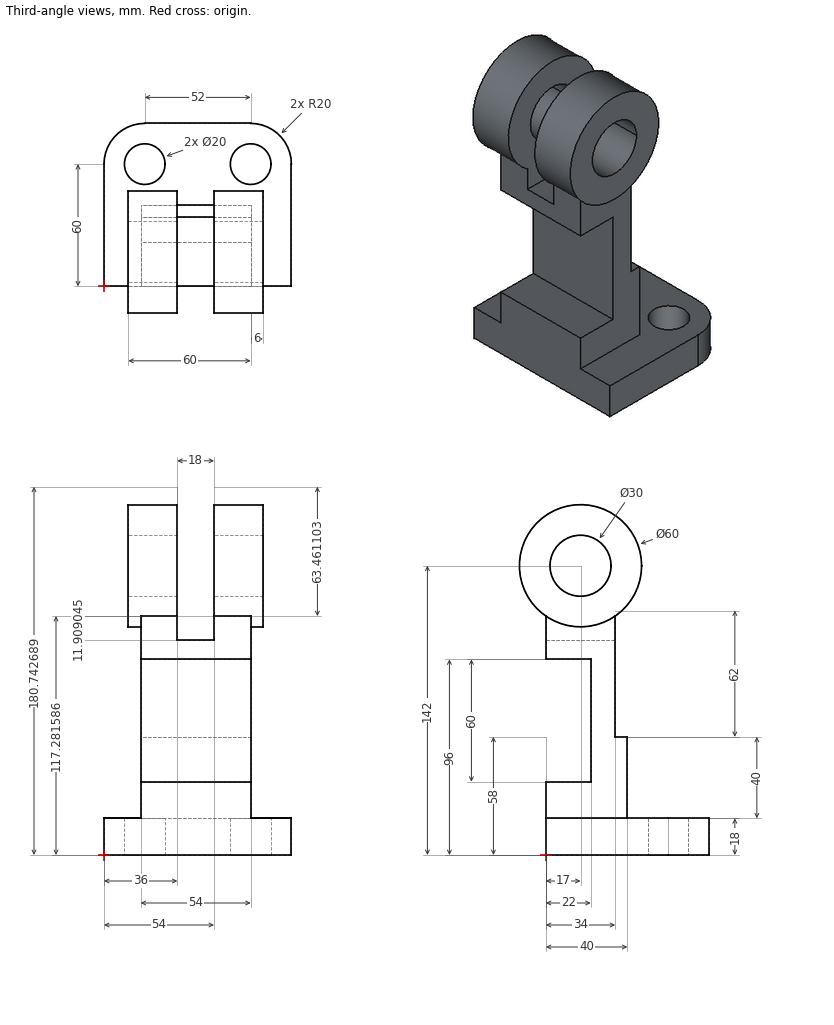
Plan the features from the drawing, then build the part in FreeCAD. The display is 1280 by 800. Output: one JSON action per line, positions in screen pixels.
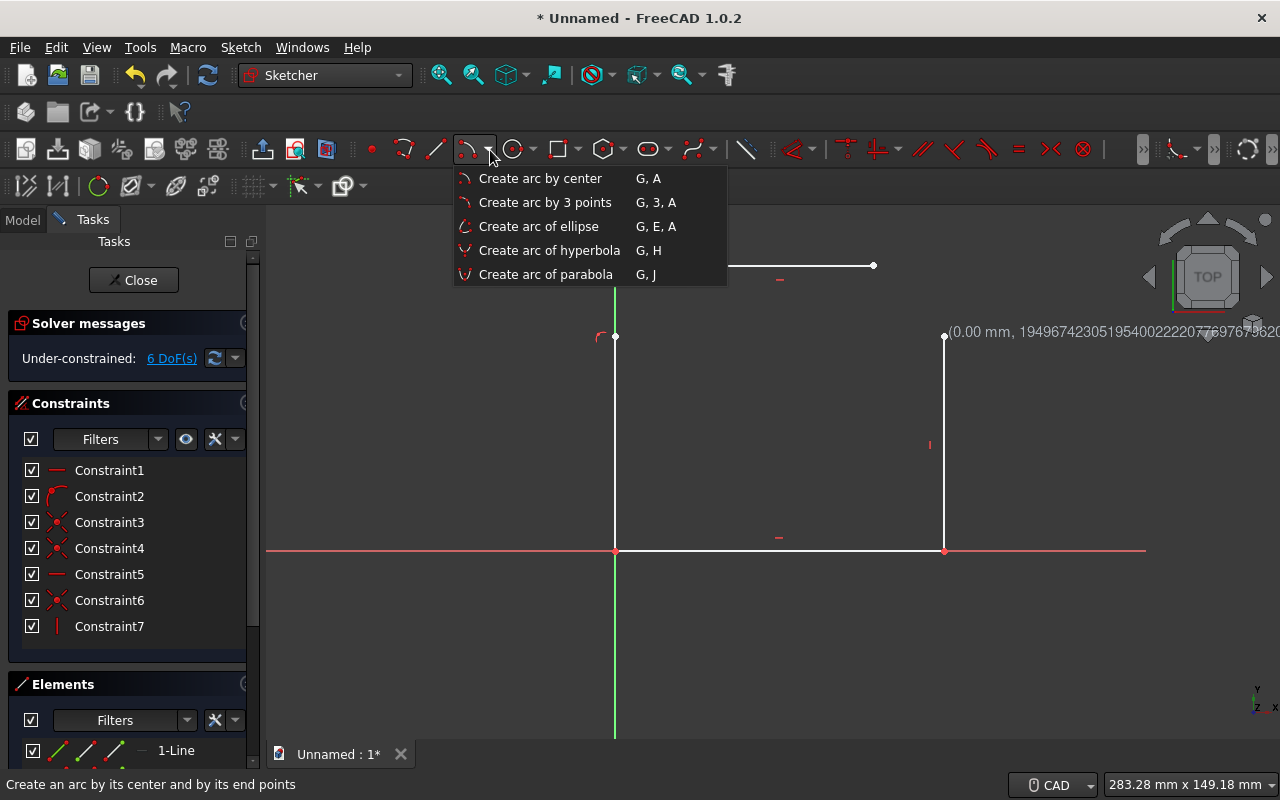
{"action": "left_click", "coordinate": [590, 202]}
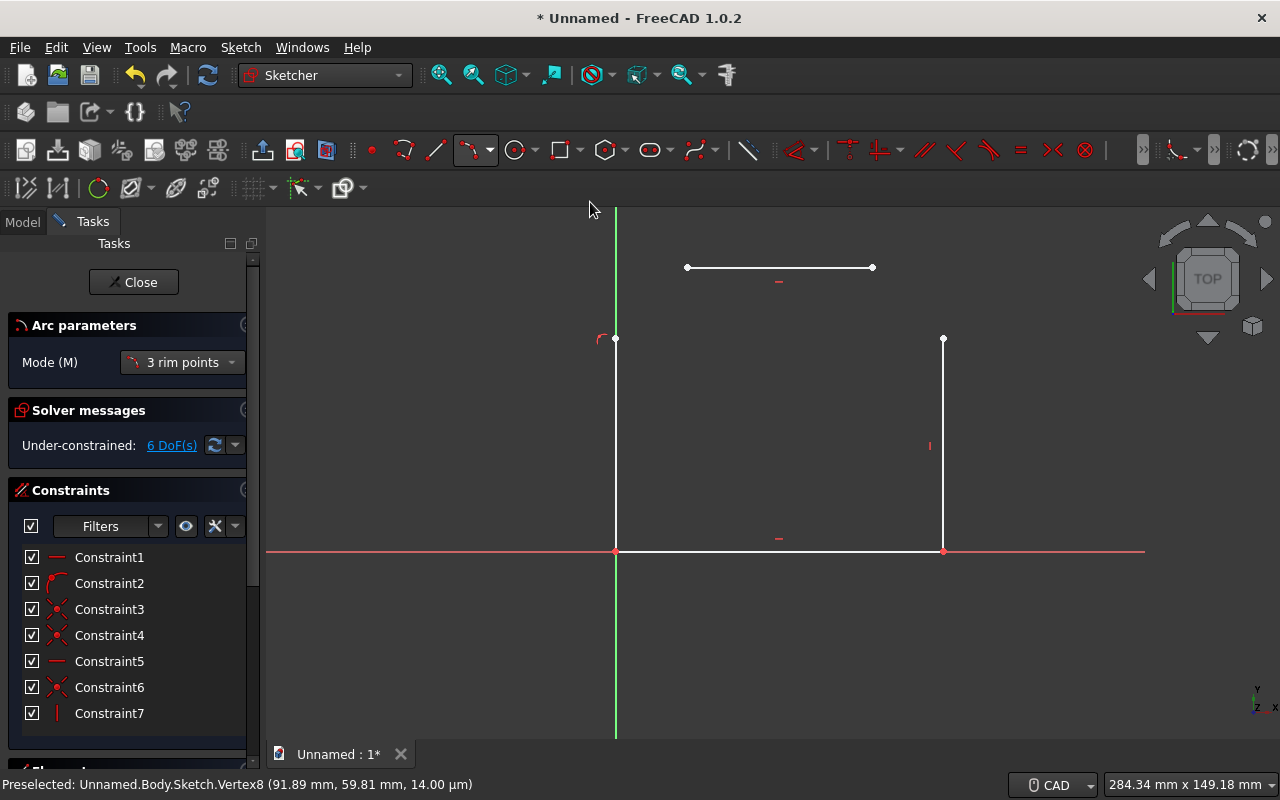
{"action": "left_click", "coordinate": [687, 268]}
{"action": "left_click", "coordinate": [616, 339]}
{"action": "left_click", "coordinate": [637, 287]}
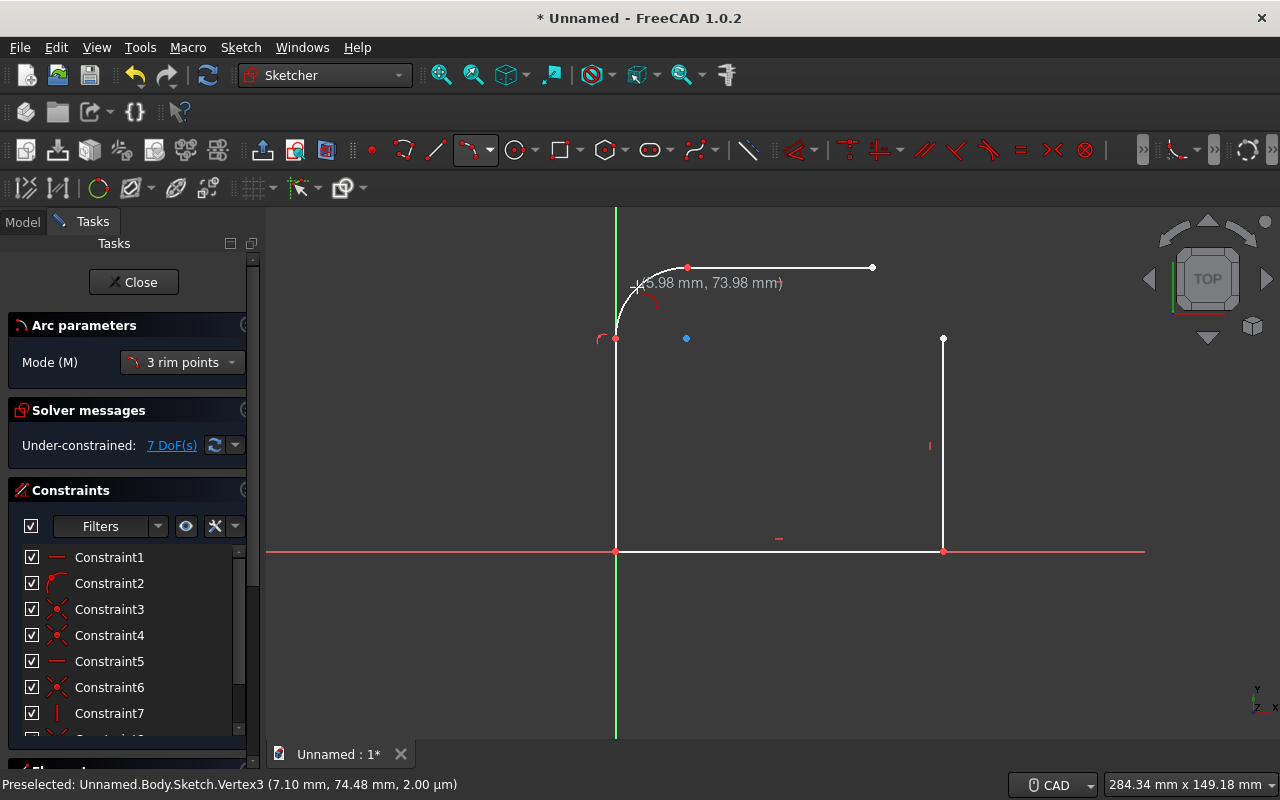
{"action": "left_click", "coordinate": [943, 339]}
{"action": "left_click", "coordinate": [873, 268]}
{"action": "left_click", "coordinate": [923, 287]}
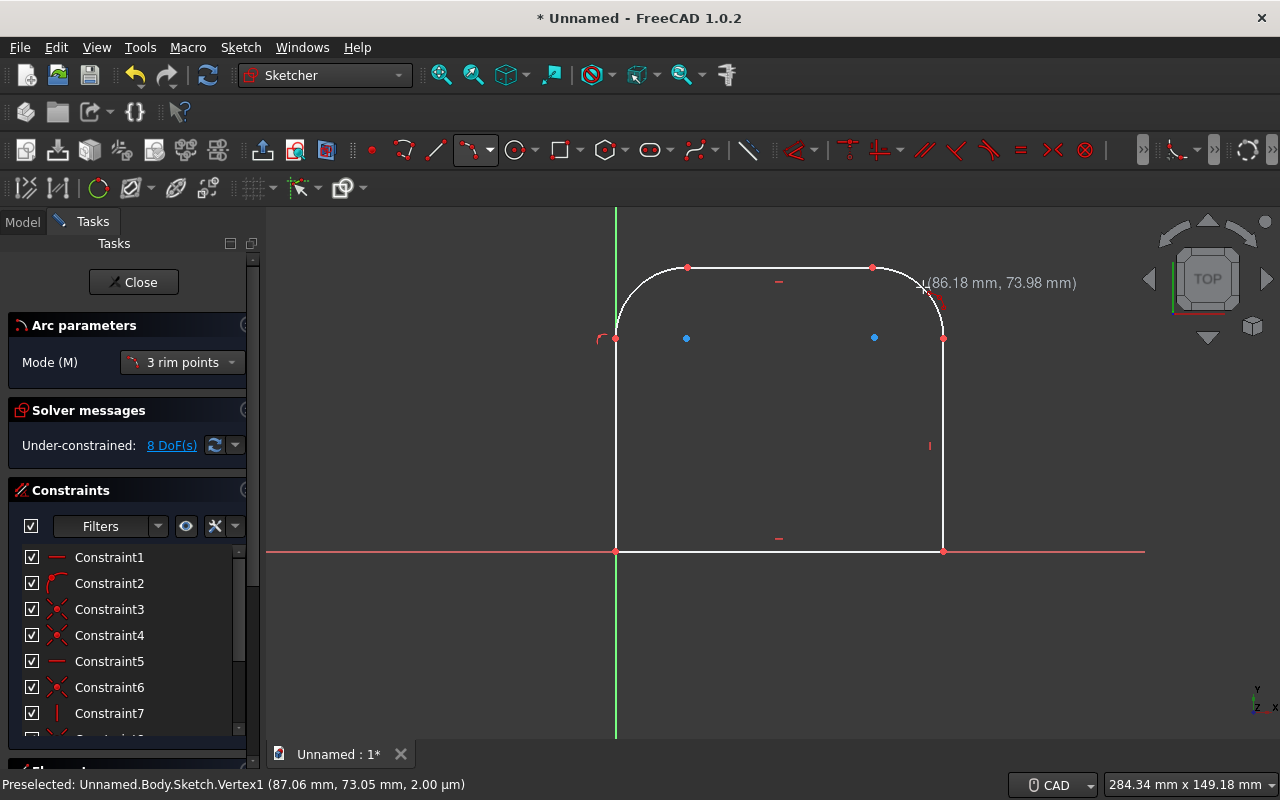
{"action": "left_click", "coordinate": [516, 150]}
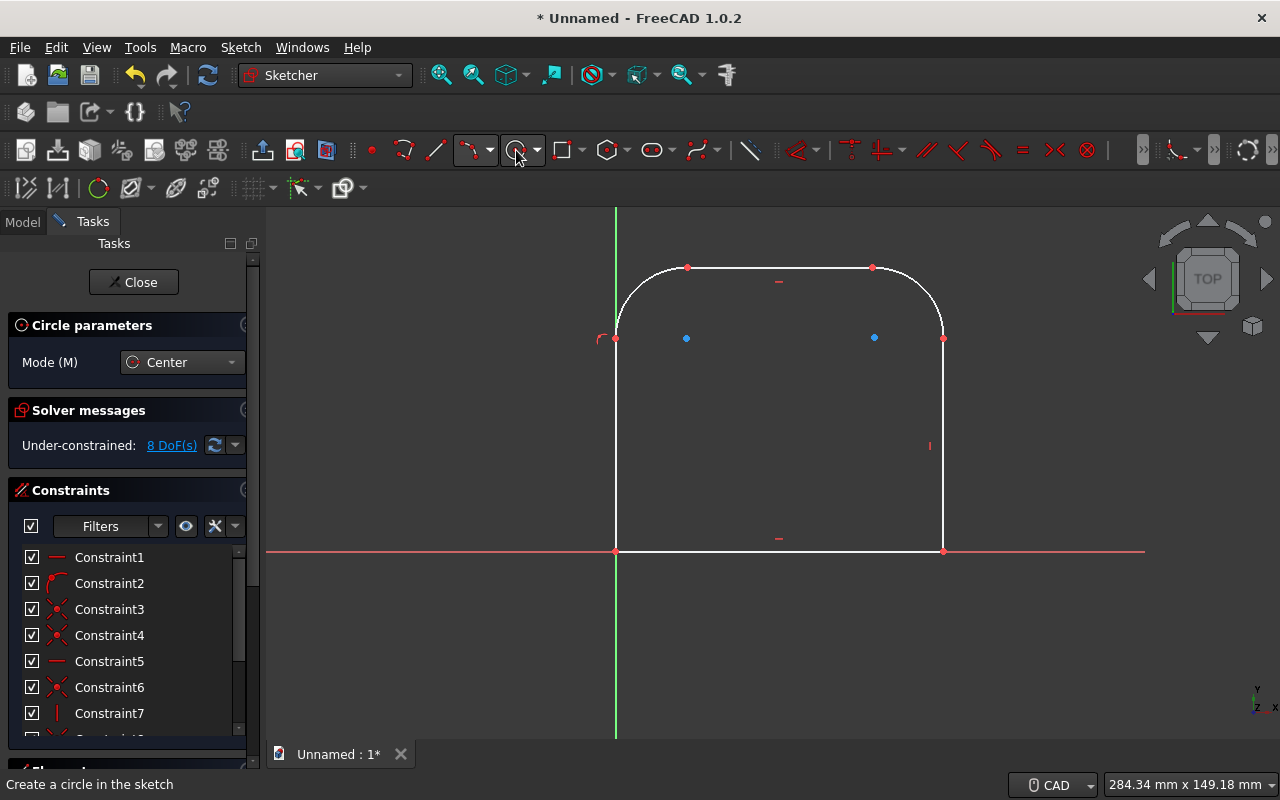
{"action": "left_click", "coordinate": [687, 338]}
{"action": "mouse_move", "coordinate": [712, 313]}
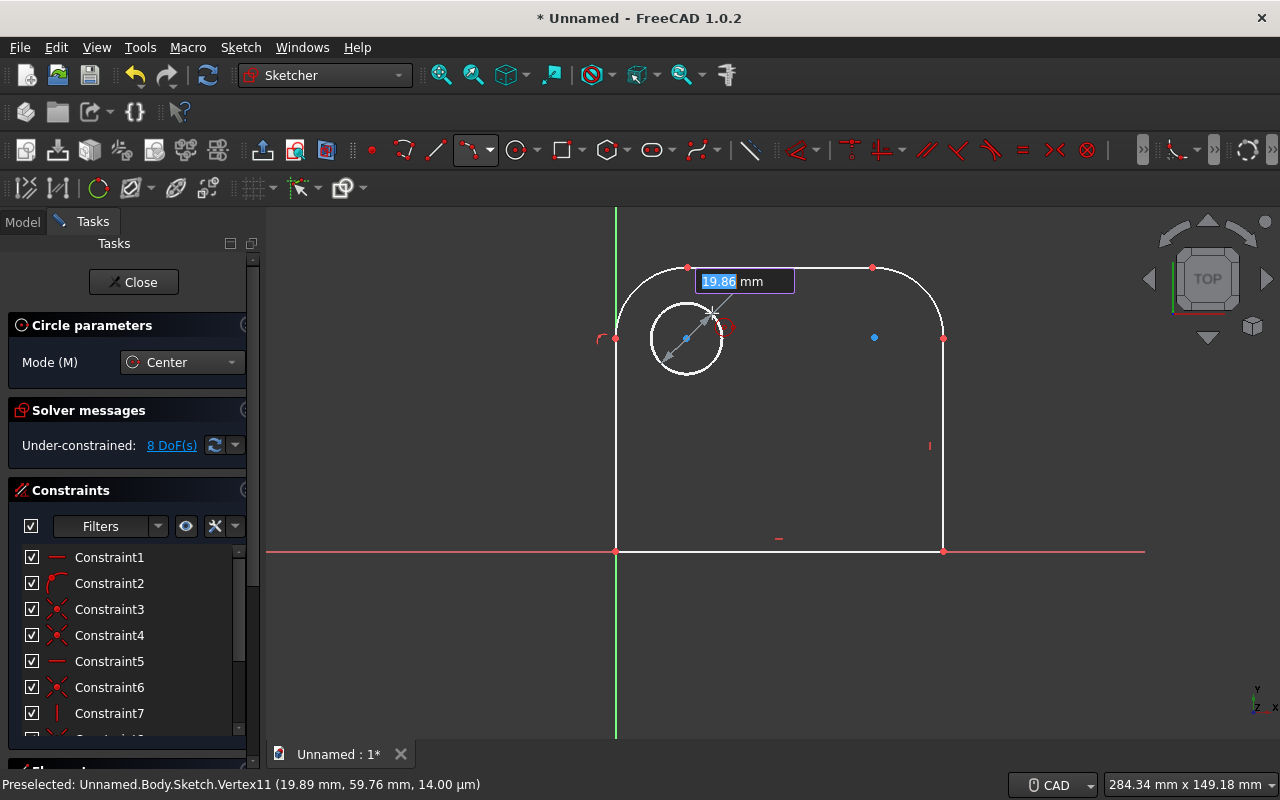
{"action": "type", "text": "20"}
{"action": "key", "text": "Return"}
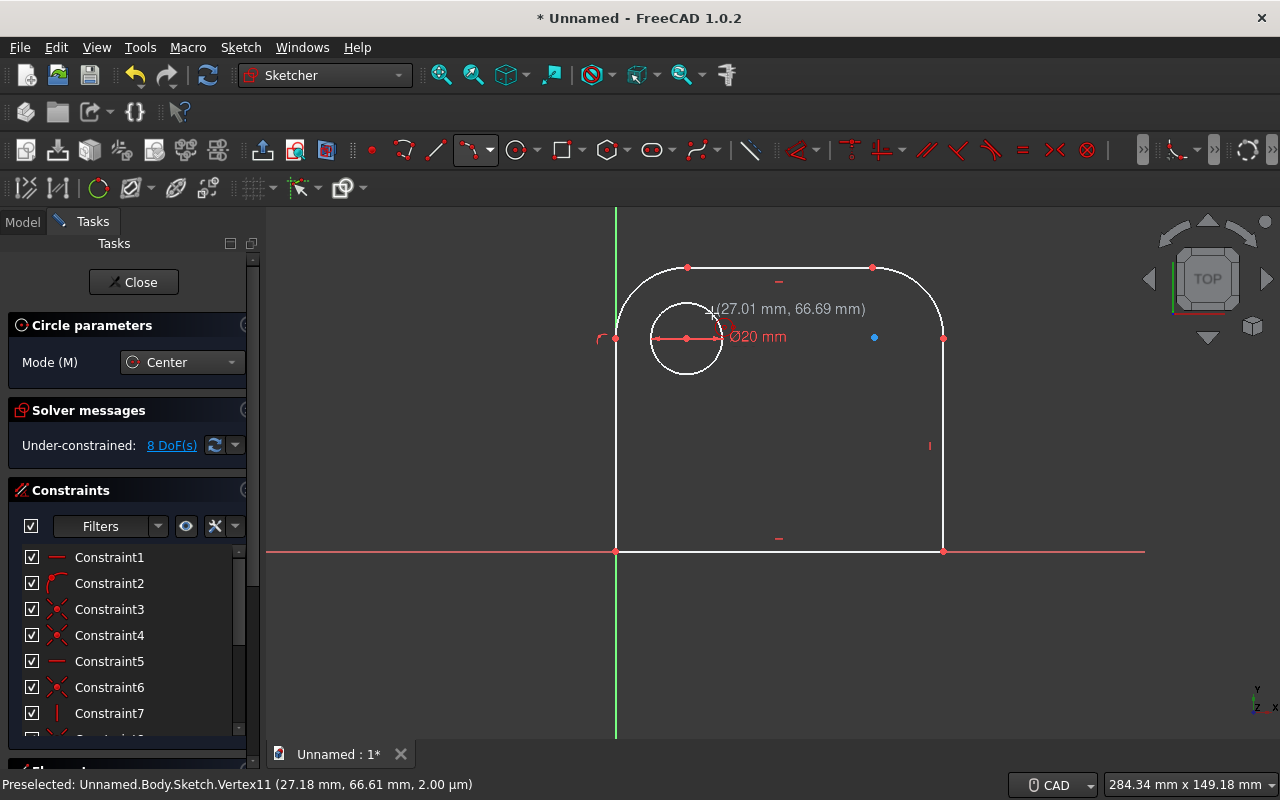
{"action": "left_click", "coordinate": [872, 338]}
{"action": "mouse_move", "coordinate": [898, 313]}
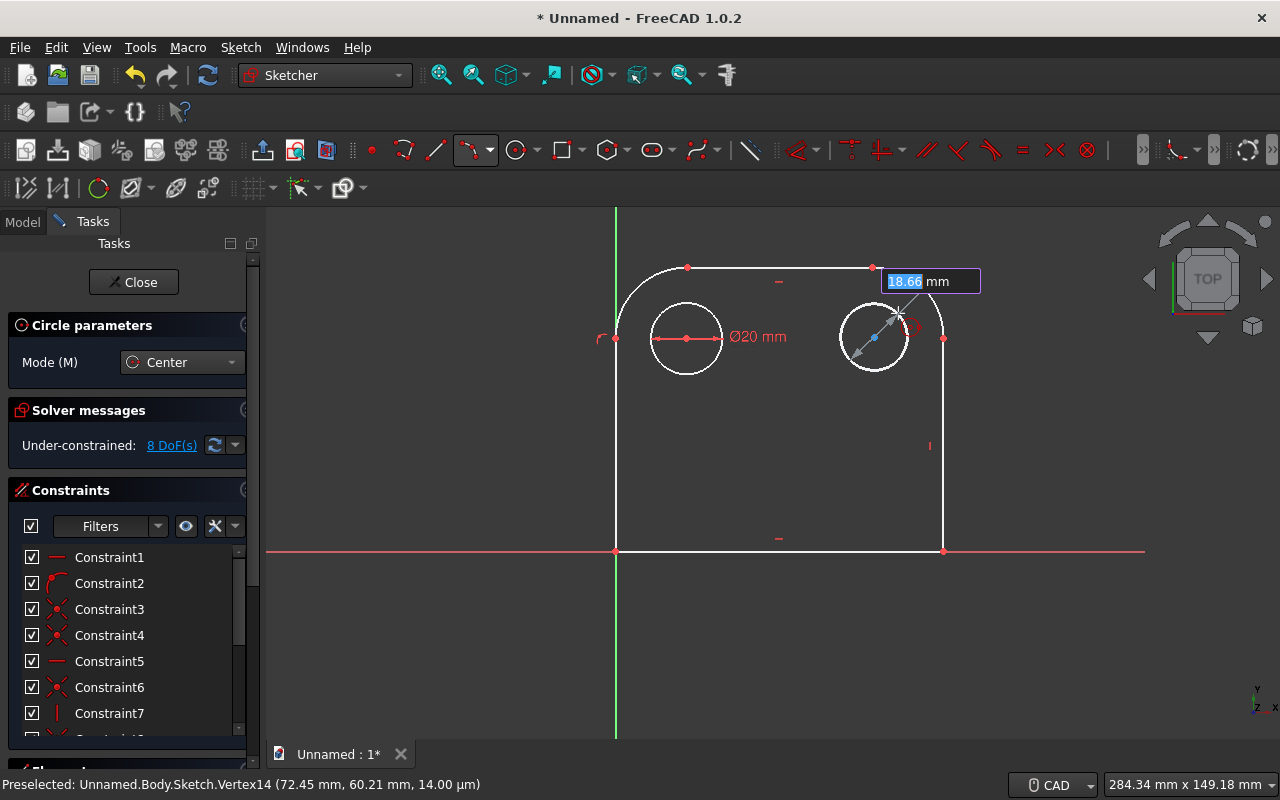
{"action": "type", "text": "20"}
{"action": "key", "text": "Return"}
{"action": "key", "text": "Escape"}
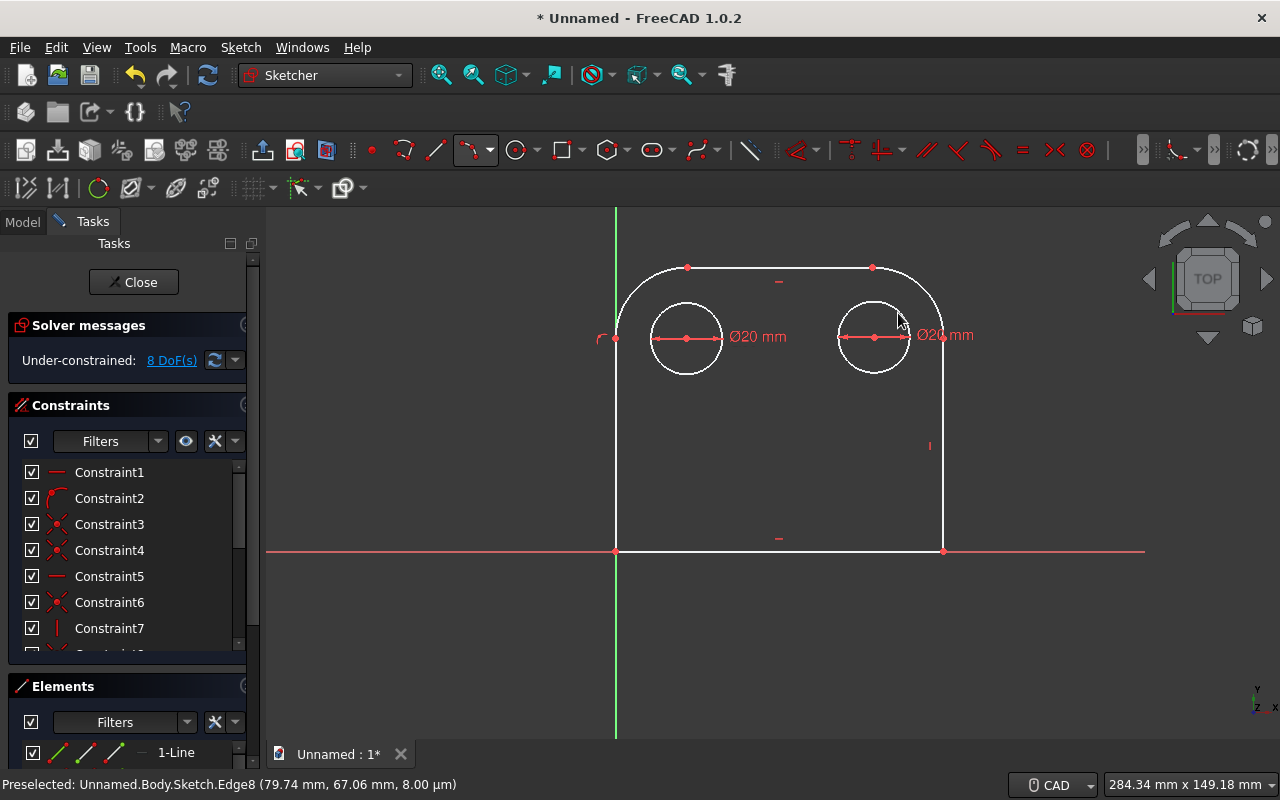
{"action": "left_click", "coordinate": [817, 268]}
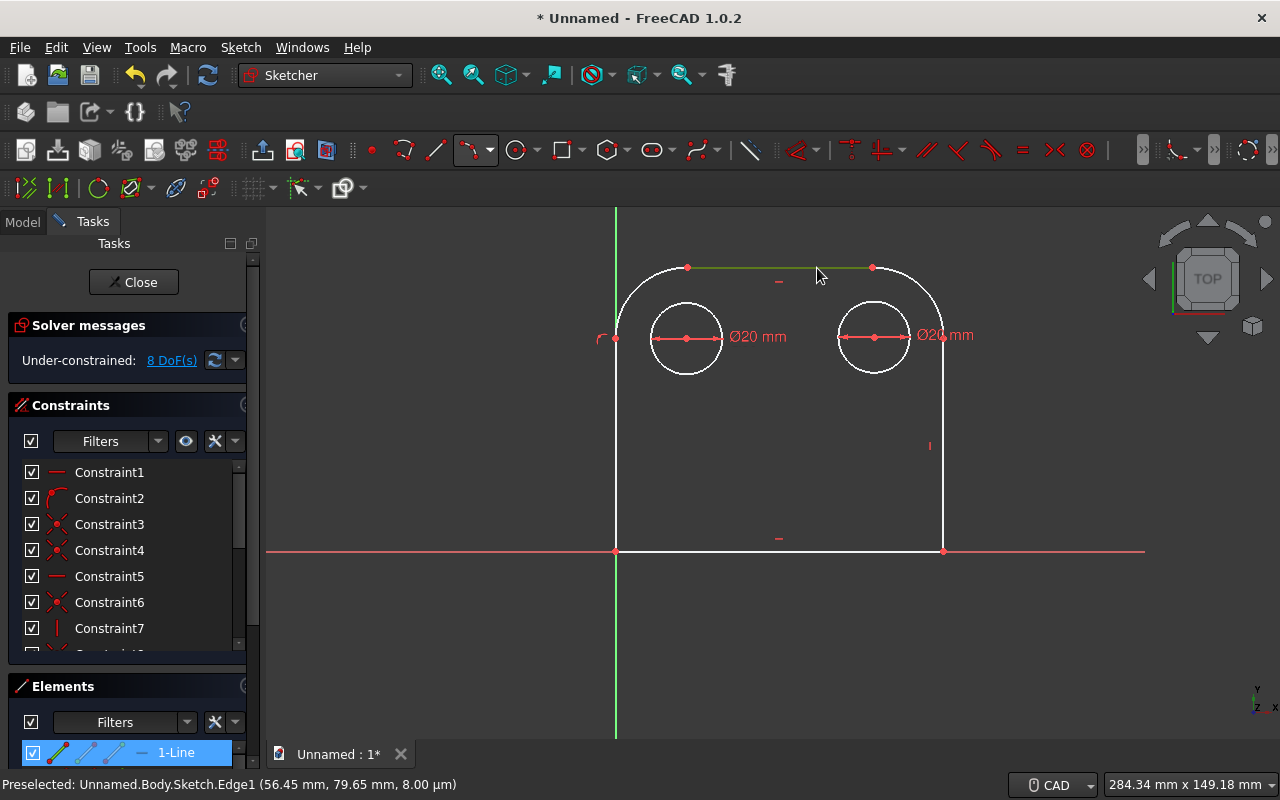
{"action": "left_click", "coordinate": [655, 275]}